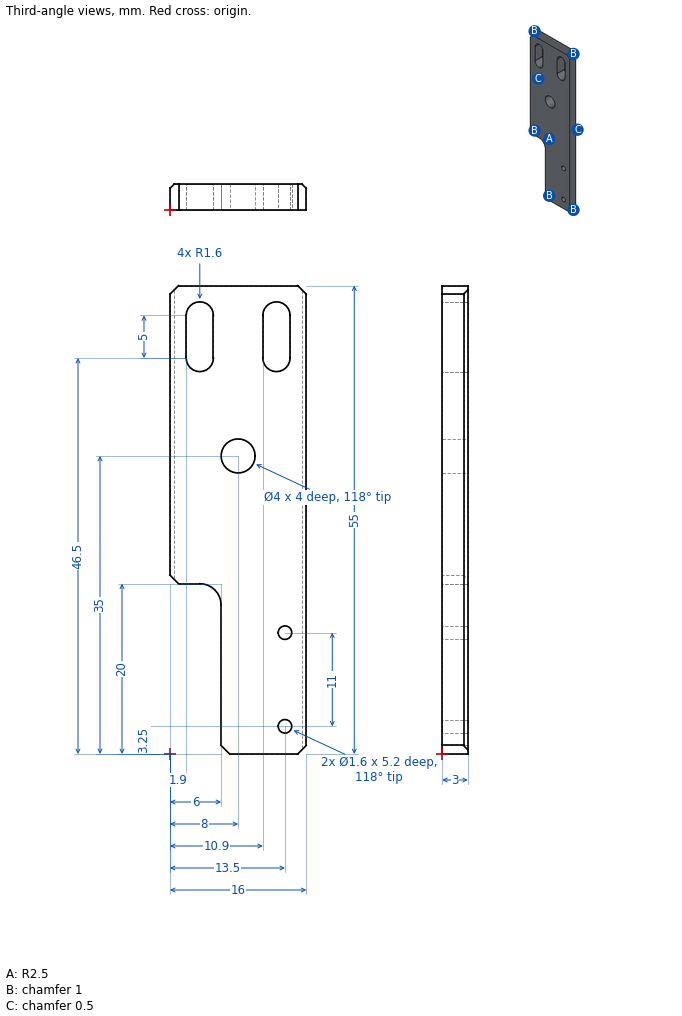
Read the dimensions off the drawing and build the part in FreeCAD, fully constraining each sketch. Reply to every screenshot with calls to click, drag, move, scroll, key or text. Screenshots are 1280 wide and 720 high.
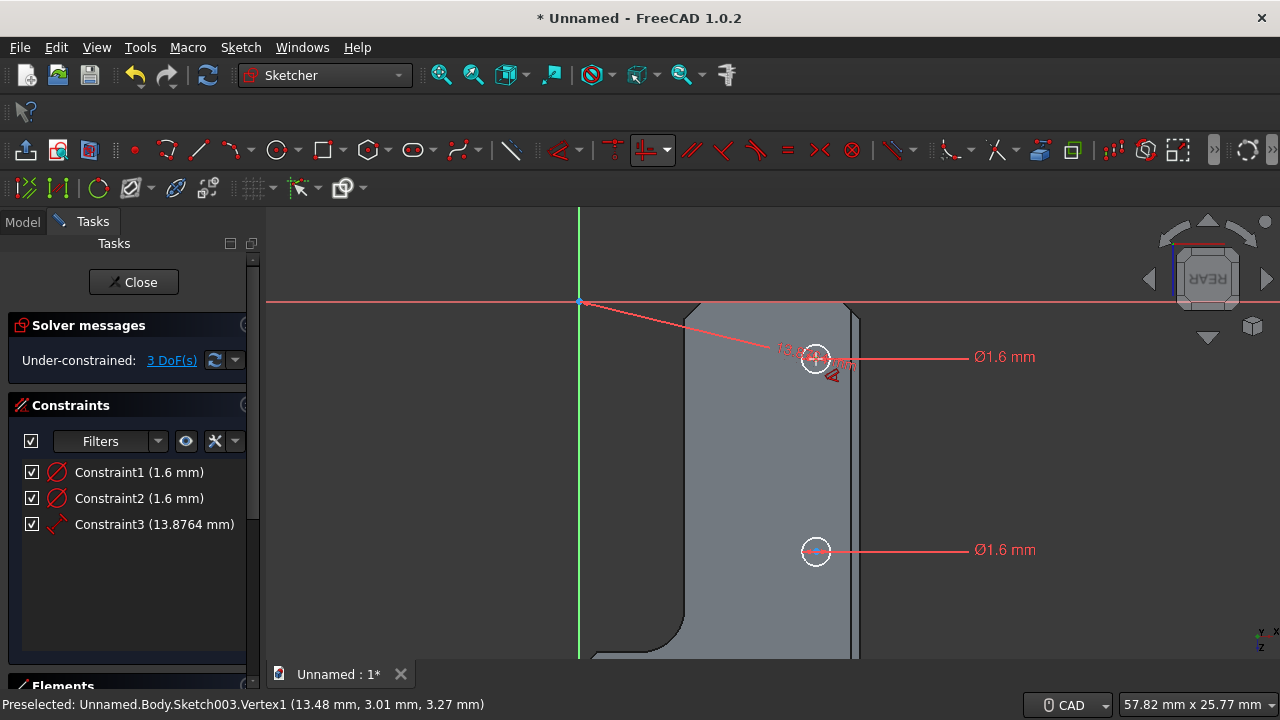
click(816, 552)
click(850, 455)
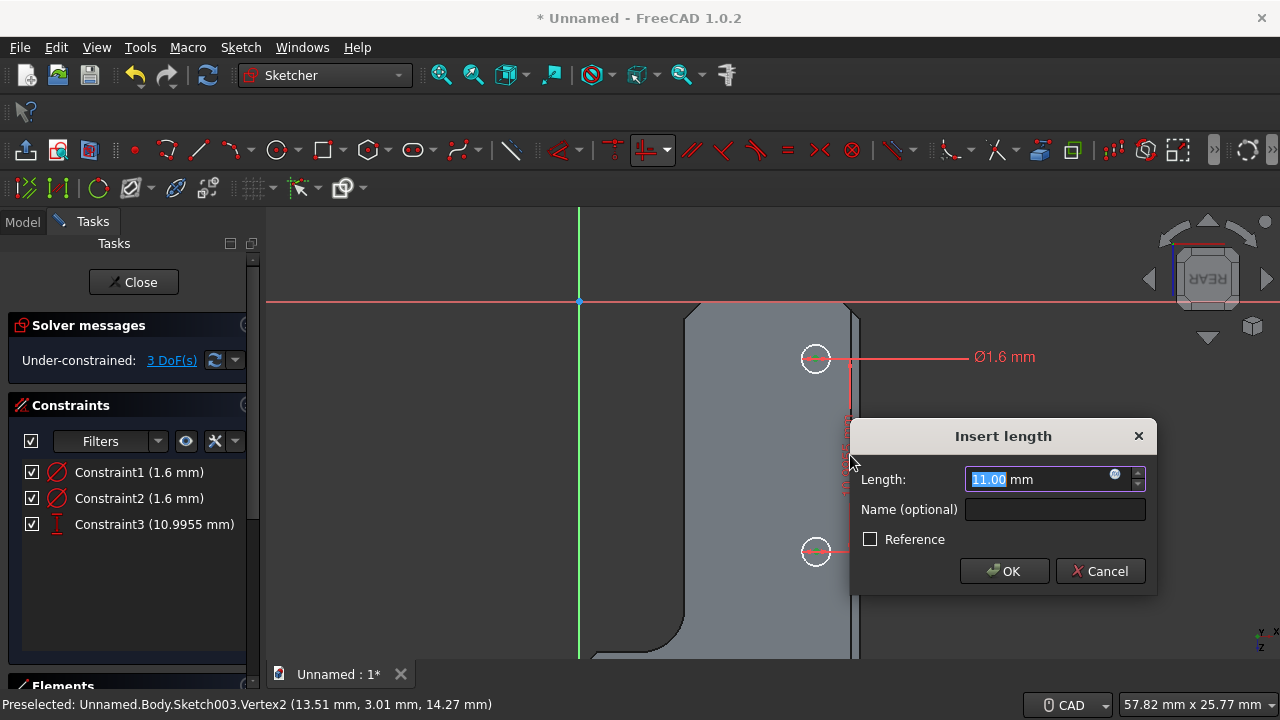
text(11)
key(Return)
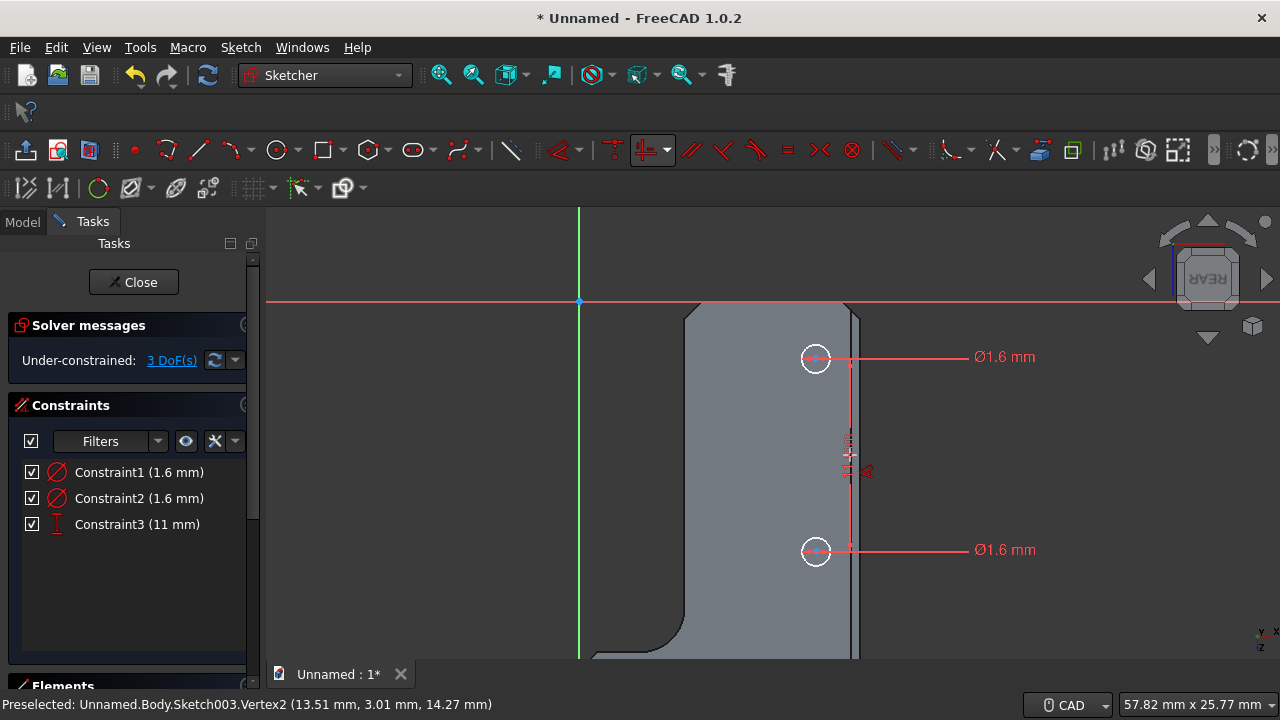
click(816, 359)
click(698, 268)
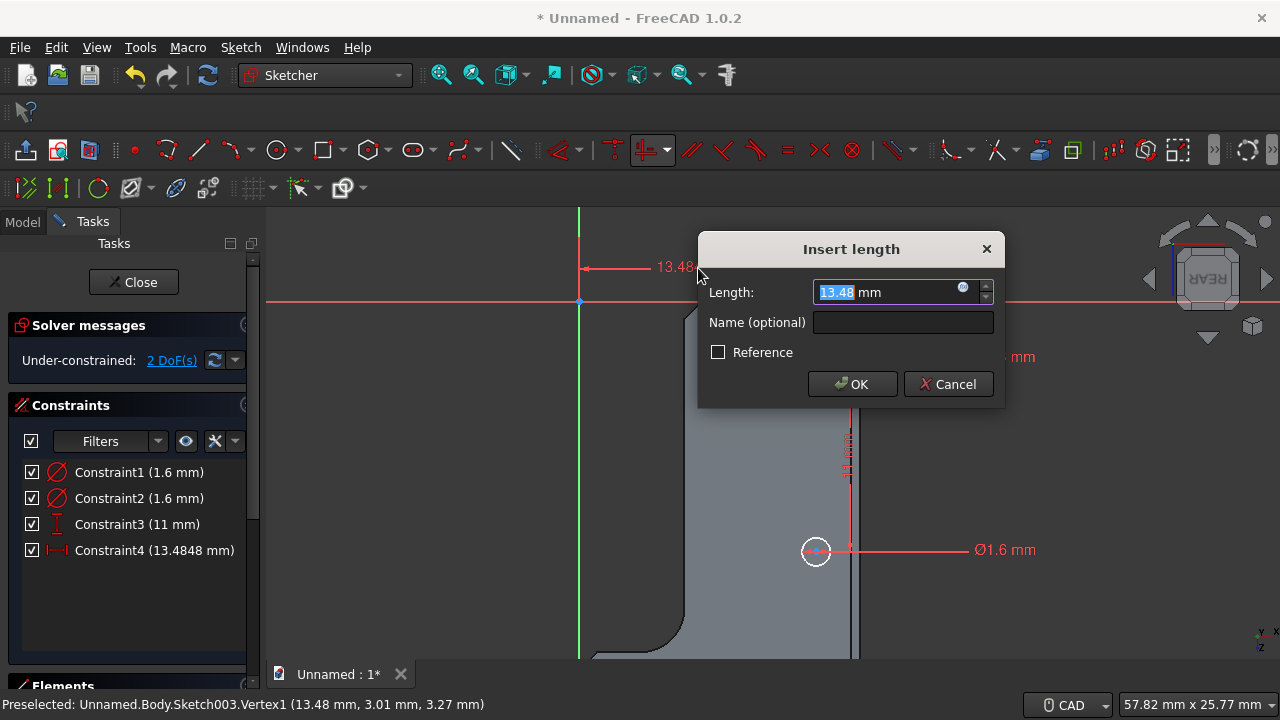
text(13.5)
key(Return)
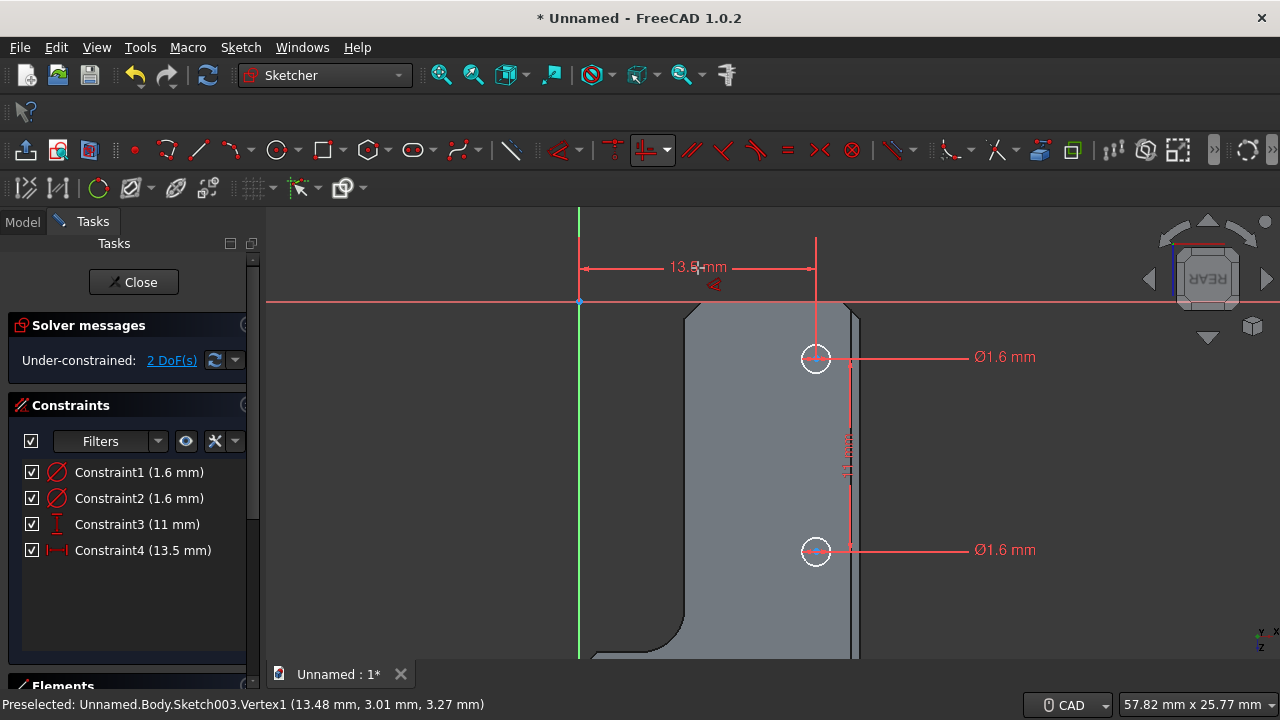
click(816, 359)
click(545, 330)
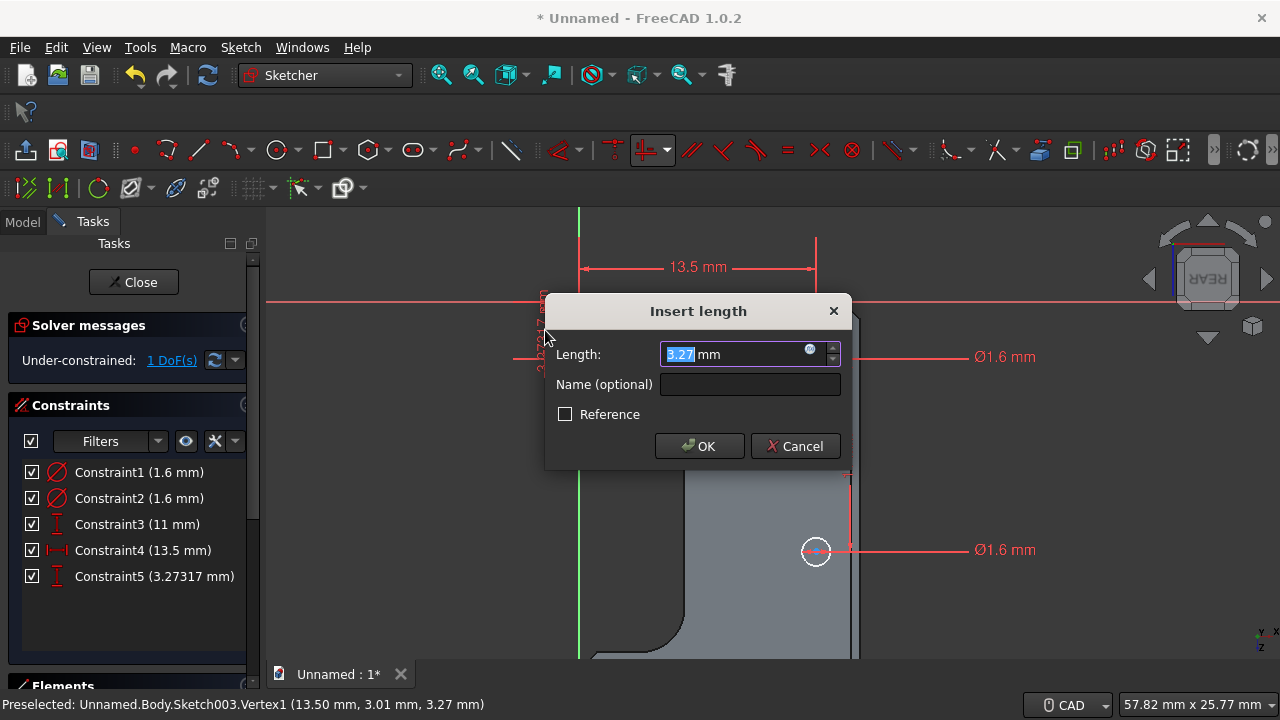
text(3.25)
key(Return)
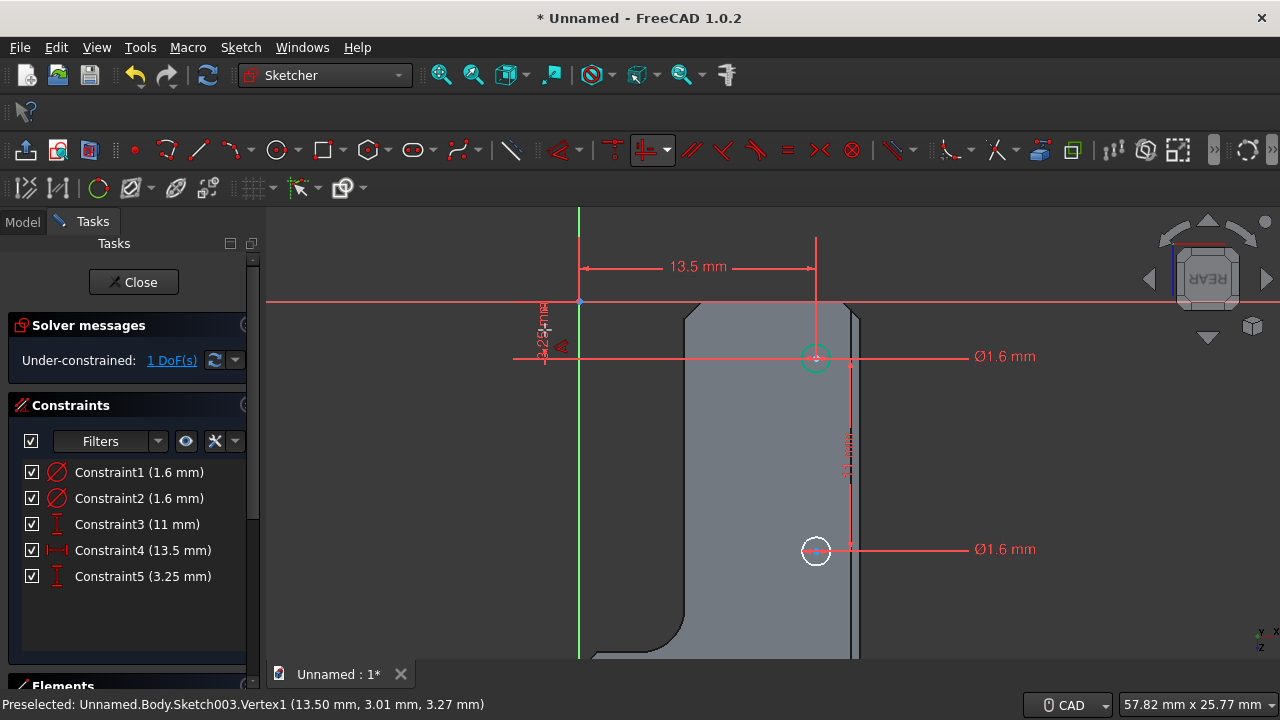
click(816, 551)
click(615, 268)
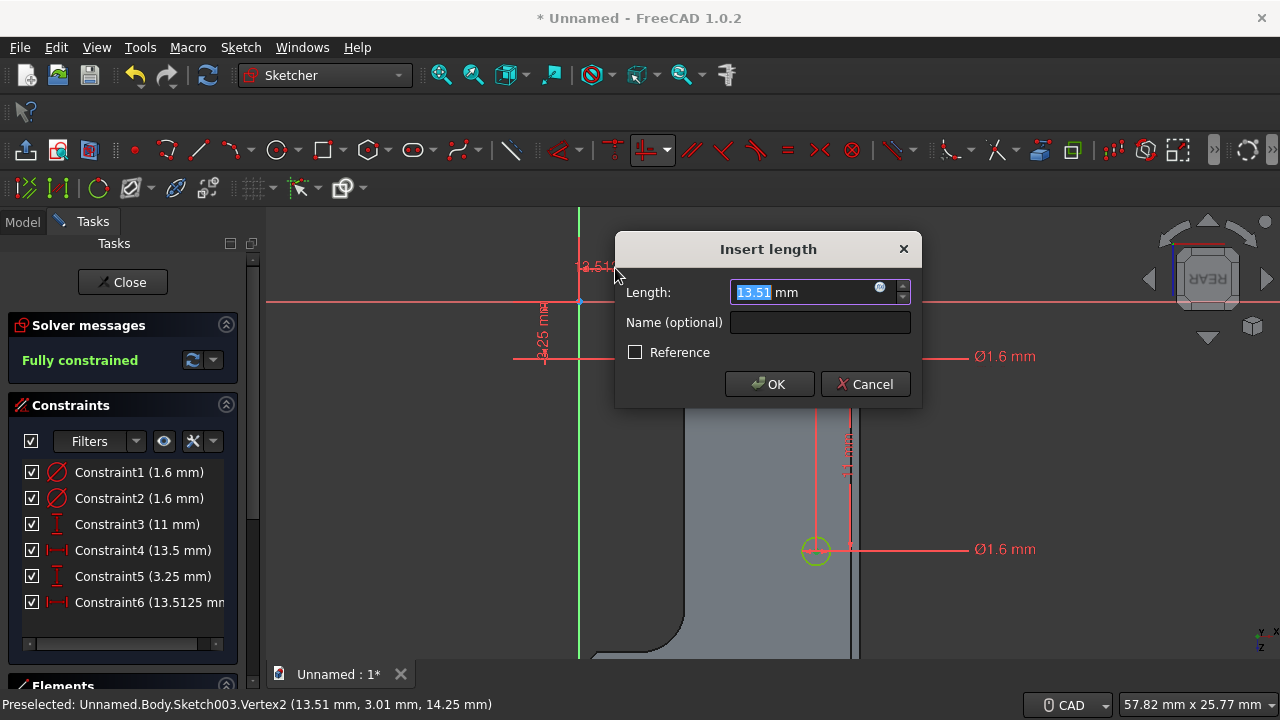
text(13.5)
key(Return)
key(Escape)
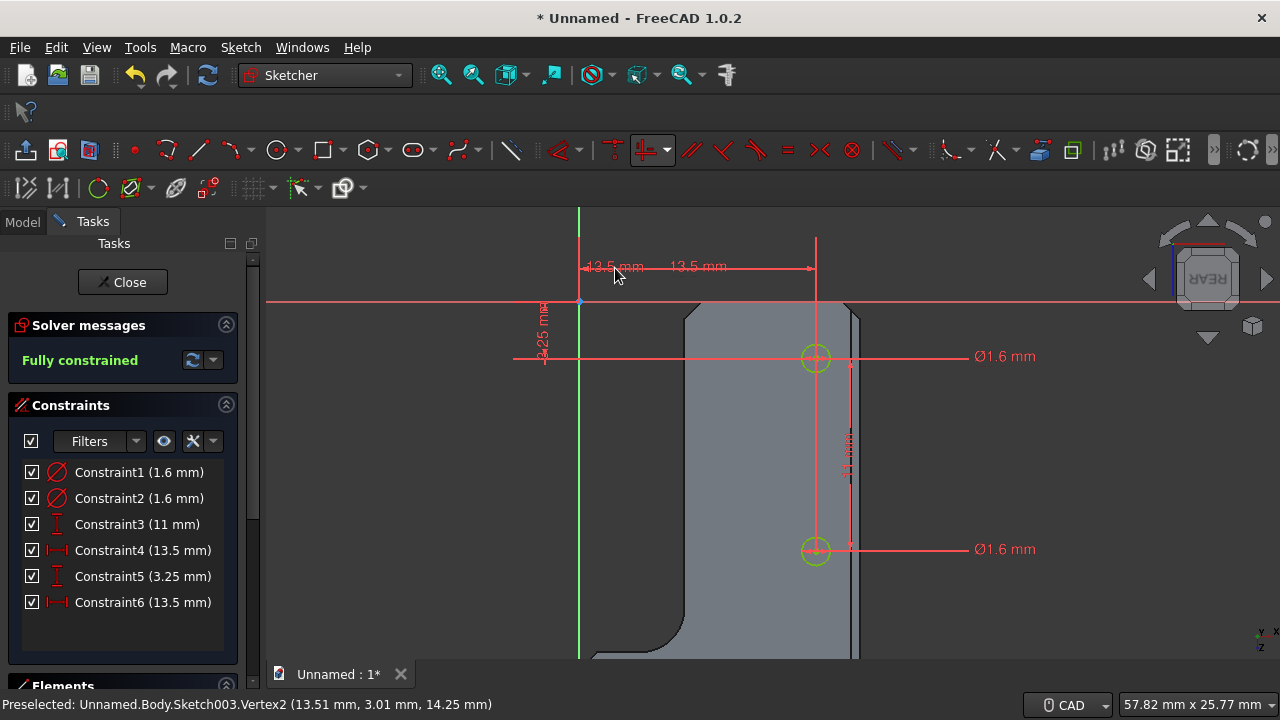
click(123, 282)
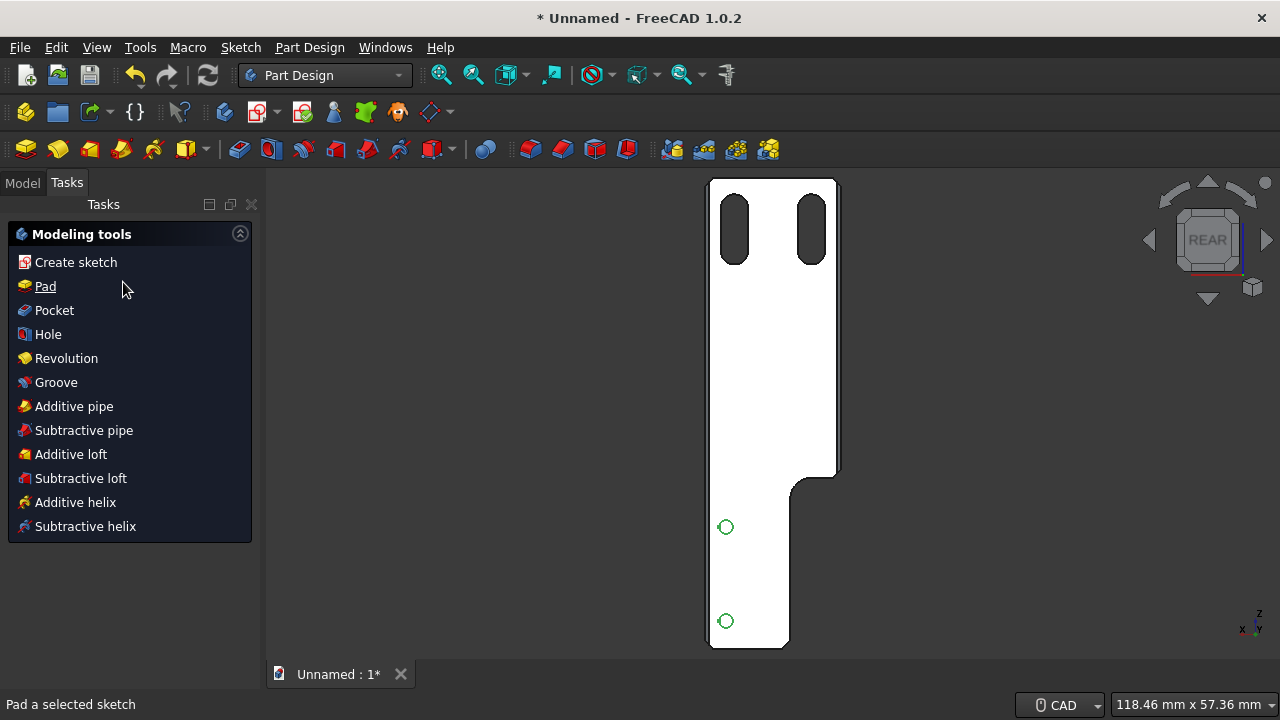
click(272, 150)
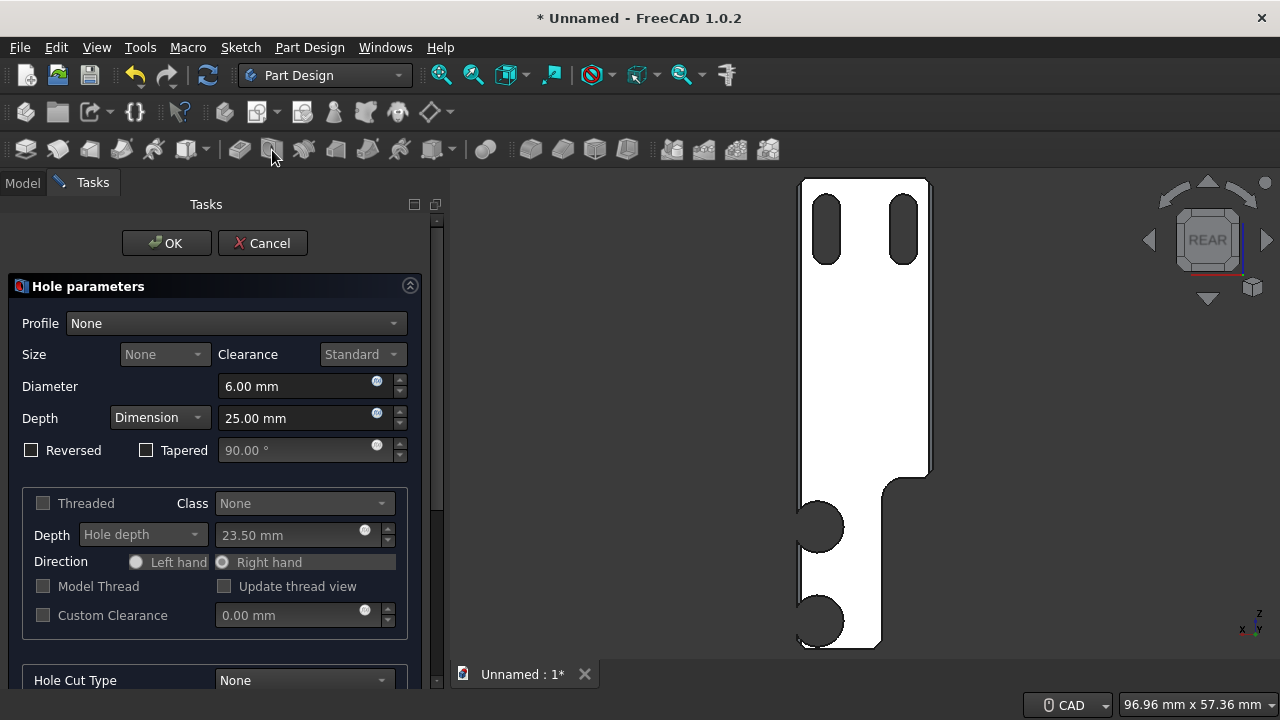
triple_click(305, 386)